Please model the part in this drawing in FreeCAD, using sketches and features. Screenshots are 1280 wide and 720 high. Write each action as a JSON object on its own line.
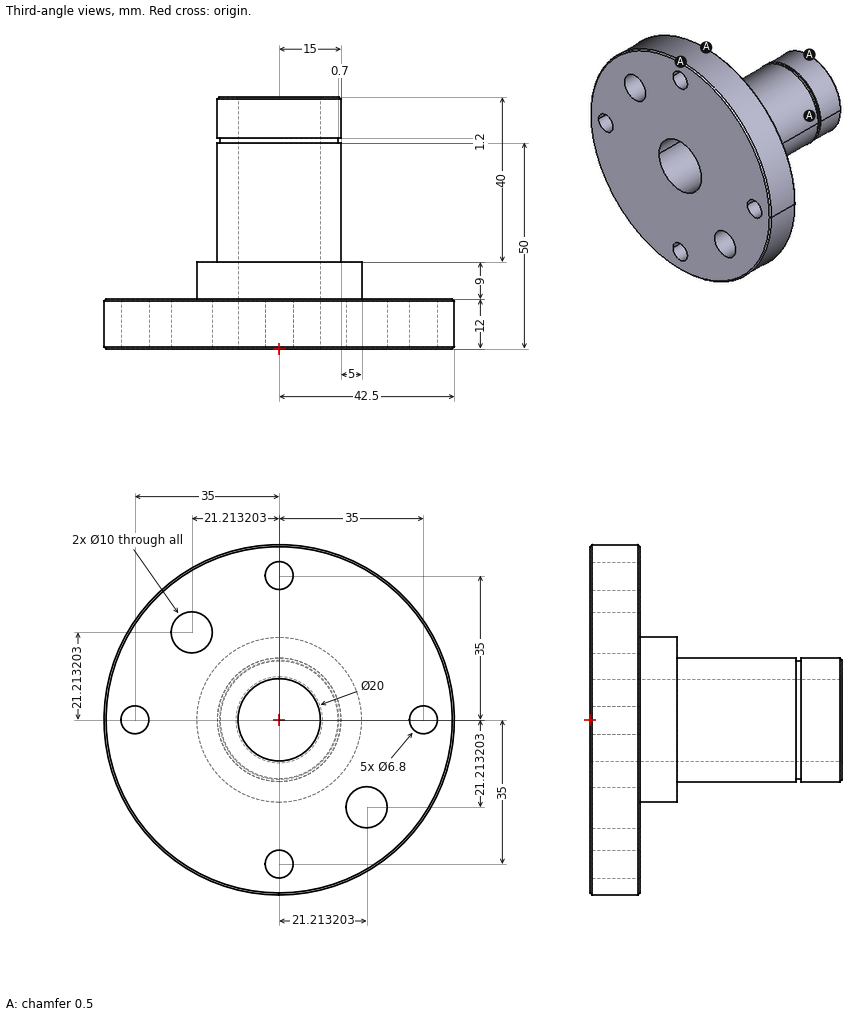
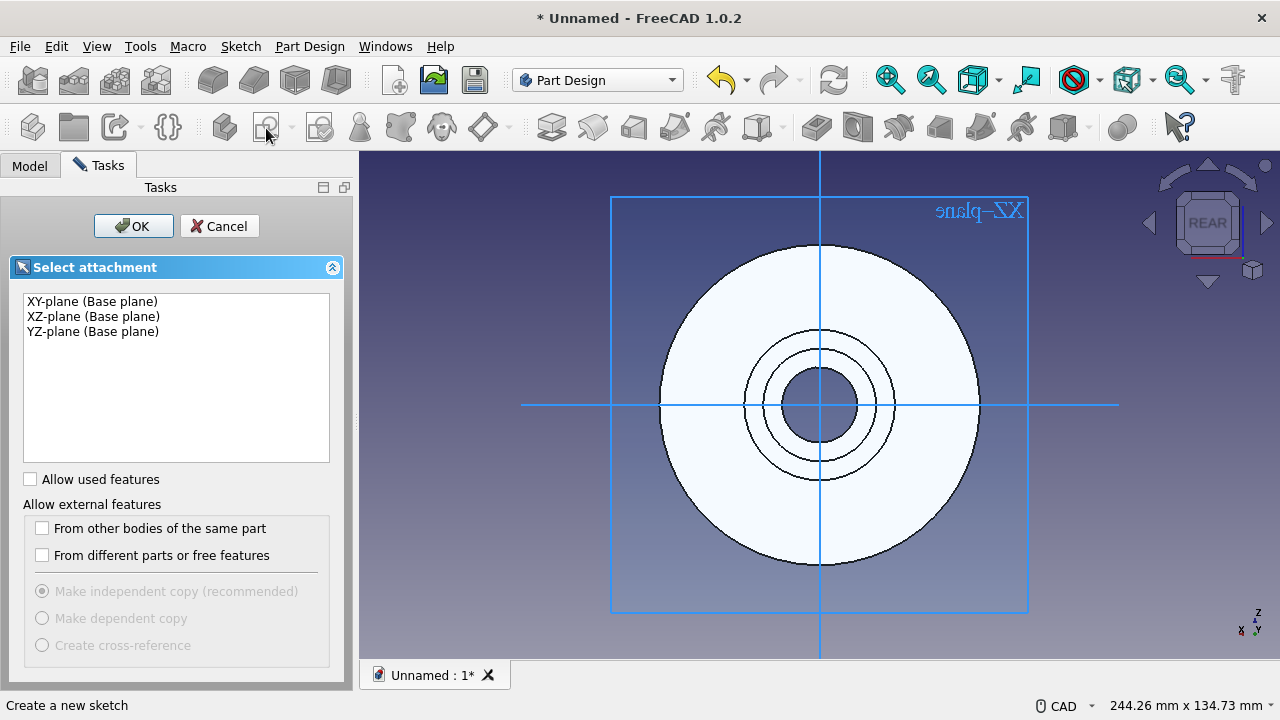
{"action": "left_click", "coordinate": [84, 302]}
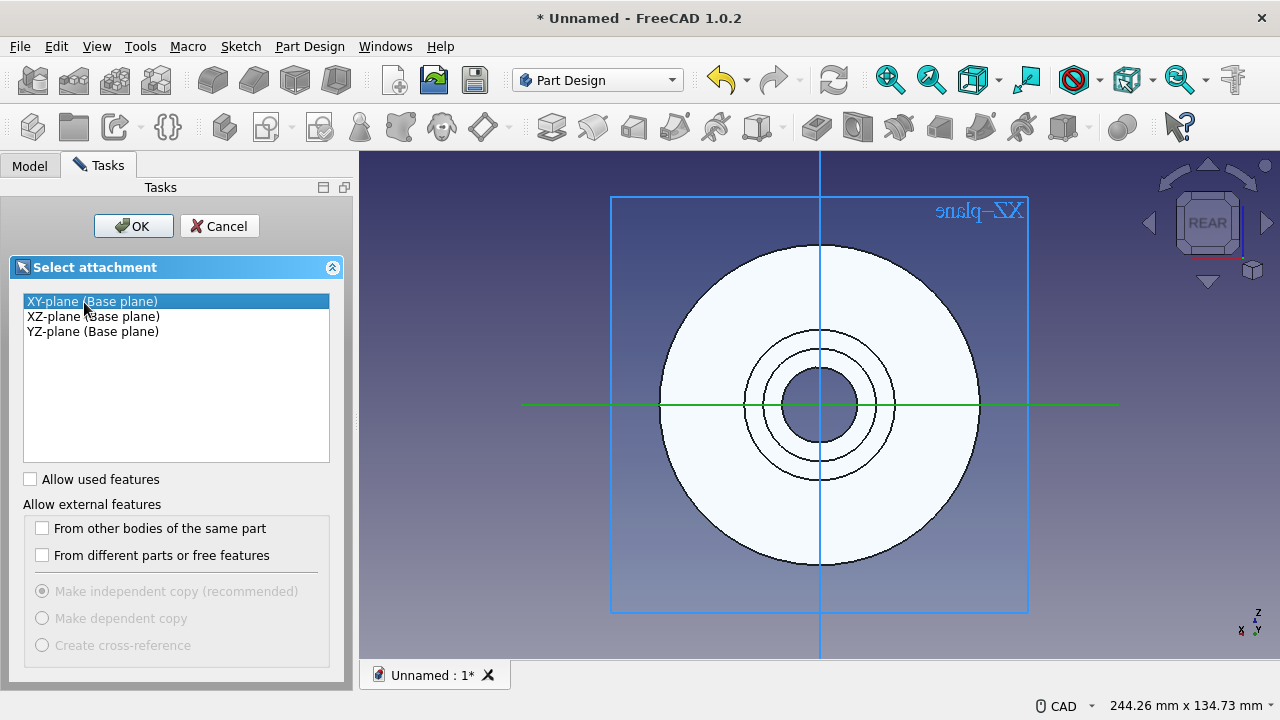
{"action": "left_click", "coordinate": [134, 226]}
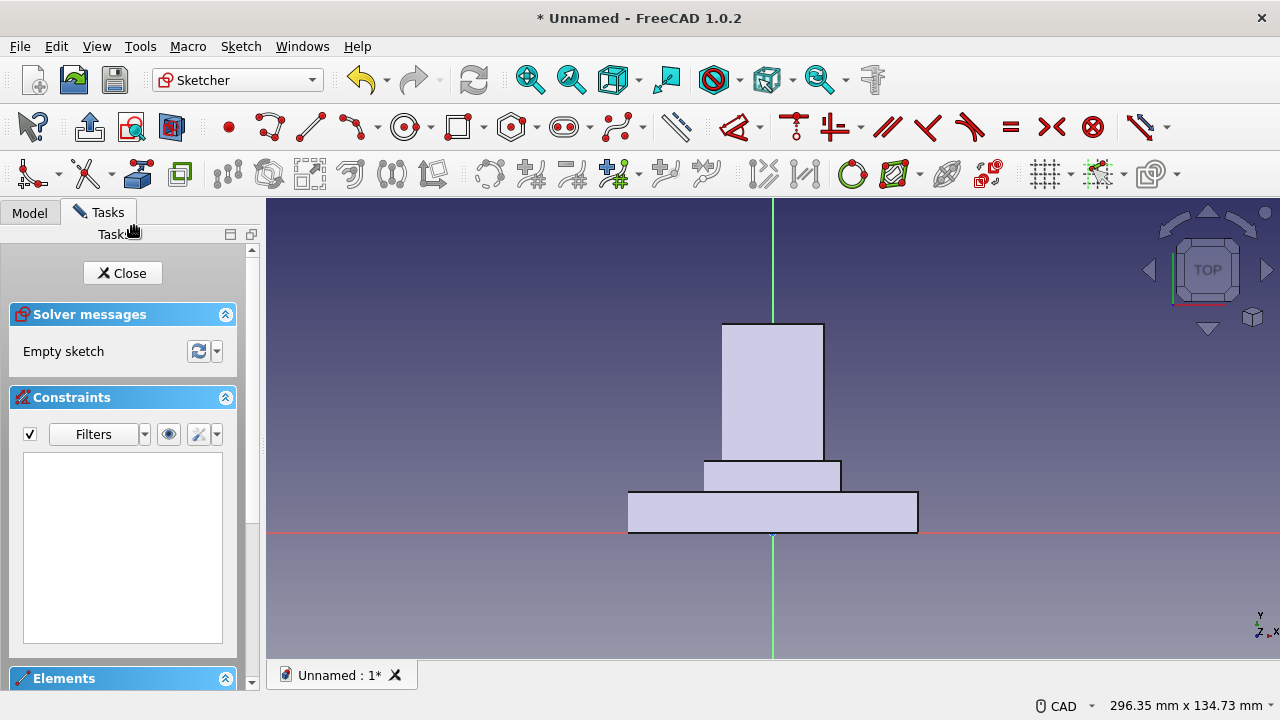
{"action": "left_click", "coordinate": [172, 128]}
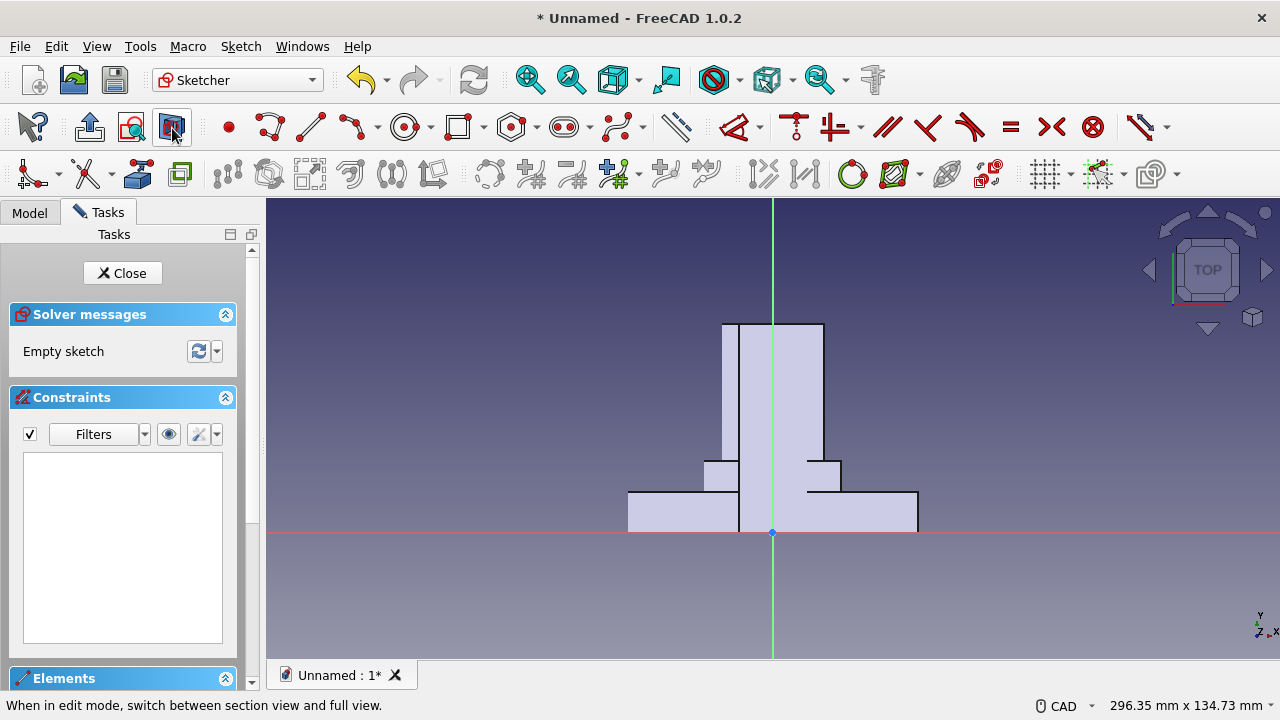
{"action": "scroll", "coordinate": [829, 356], "scroll_direction": "up", "scroll_amount": 15}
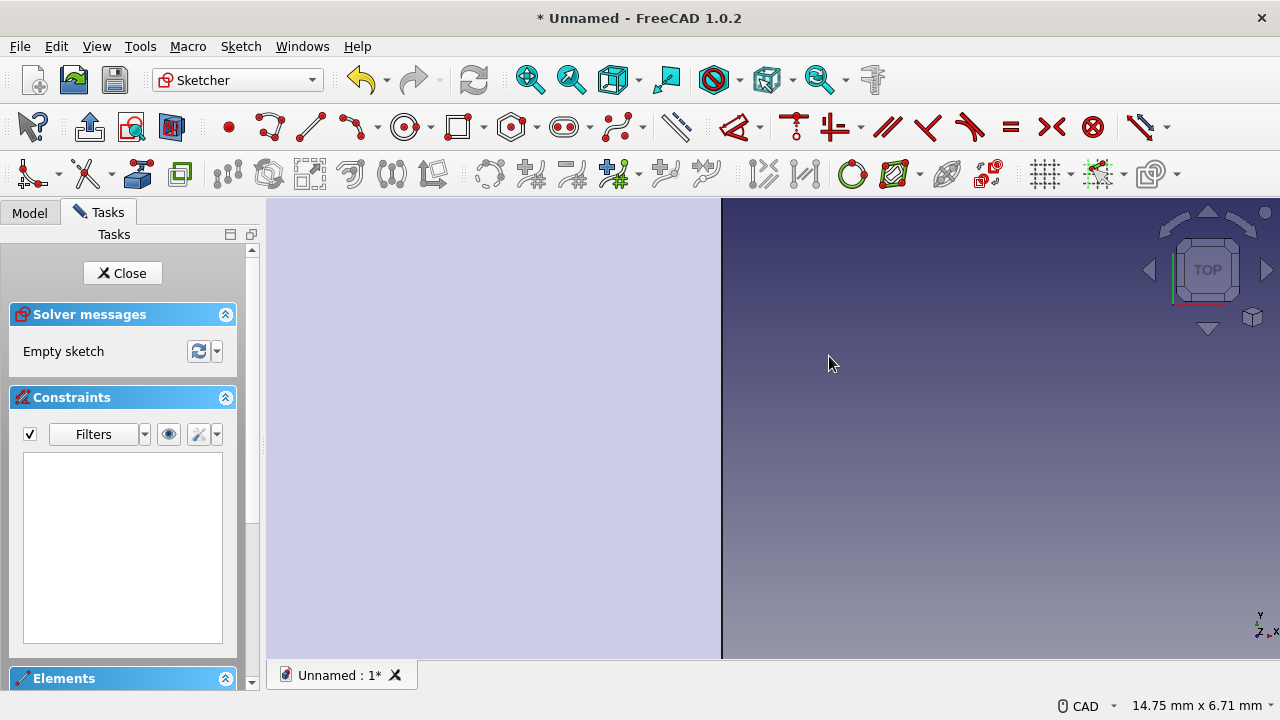
{"action": "scroll", "coordinate": [695, 422], "scroll_direction": "up", "scroll_amount": 6}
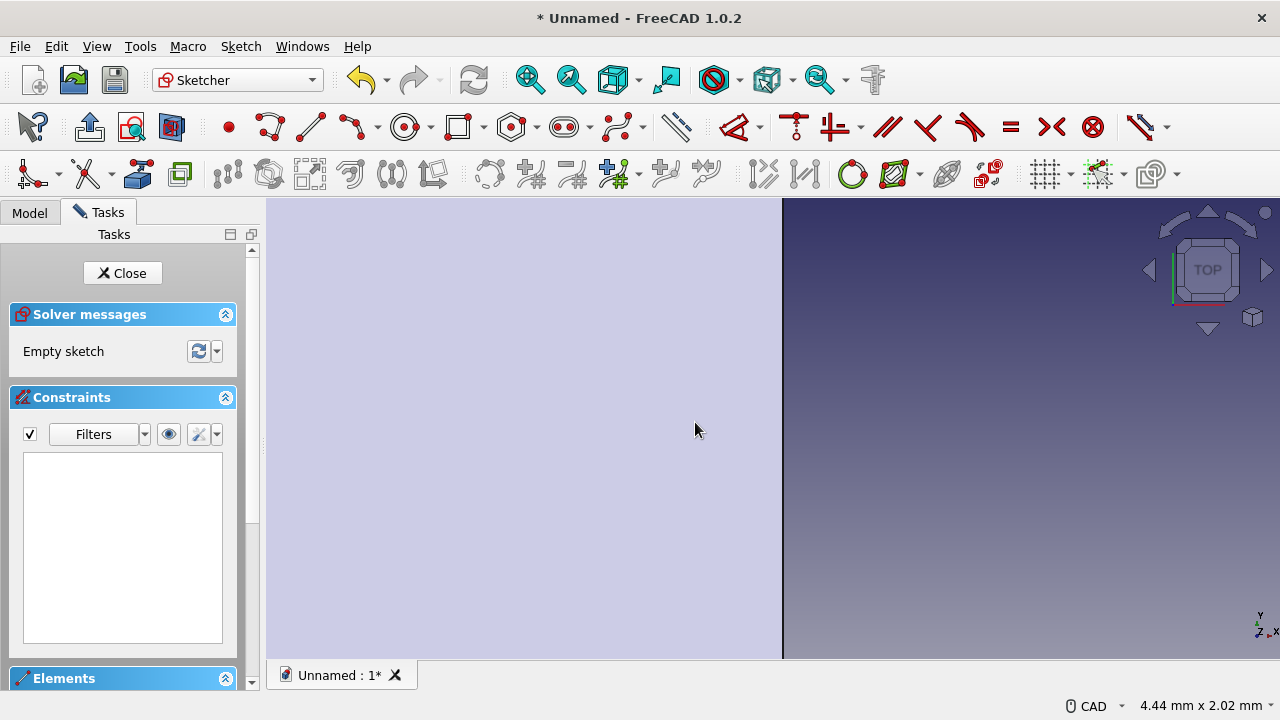
{"action": "key", "text": "g r"}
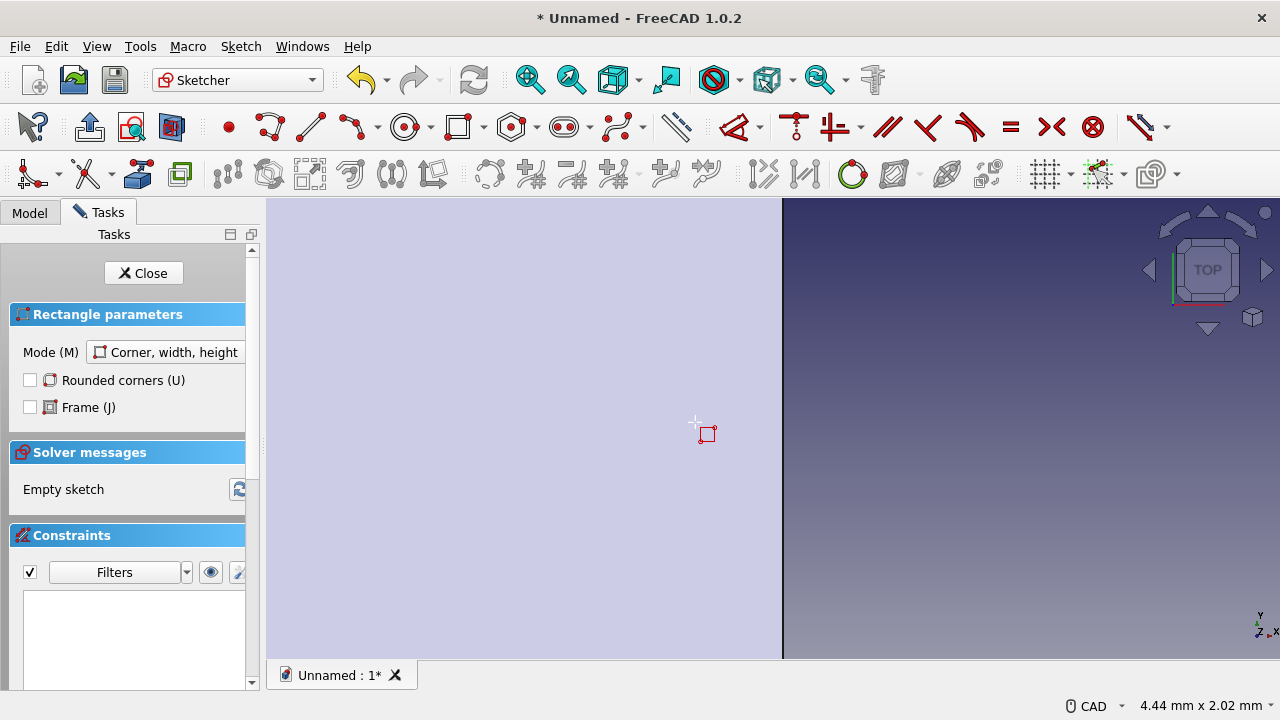
{"action": "left_click", "coordinate": [624, 291]}
{"action": "left_click", "coordinate": [783, 565]}
{"action": "key", "text": "Escape"}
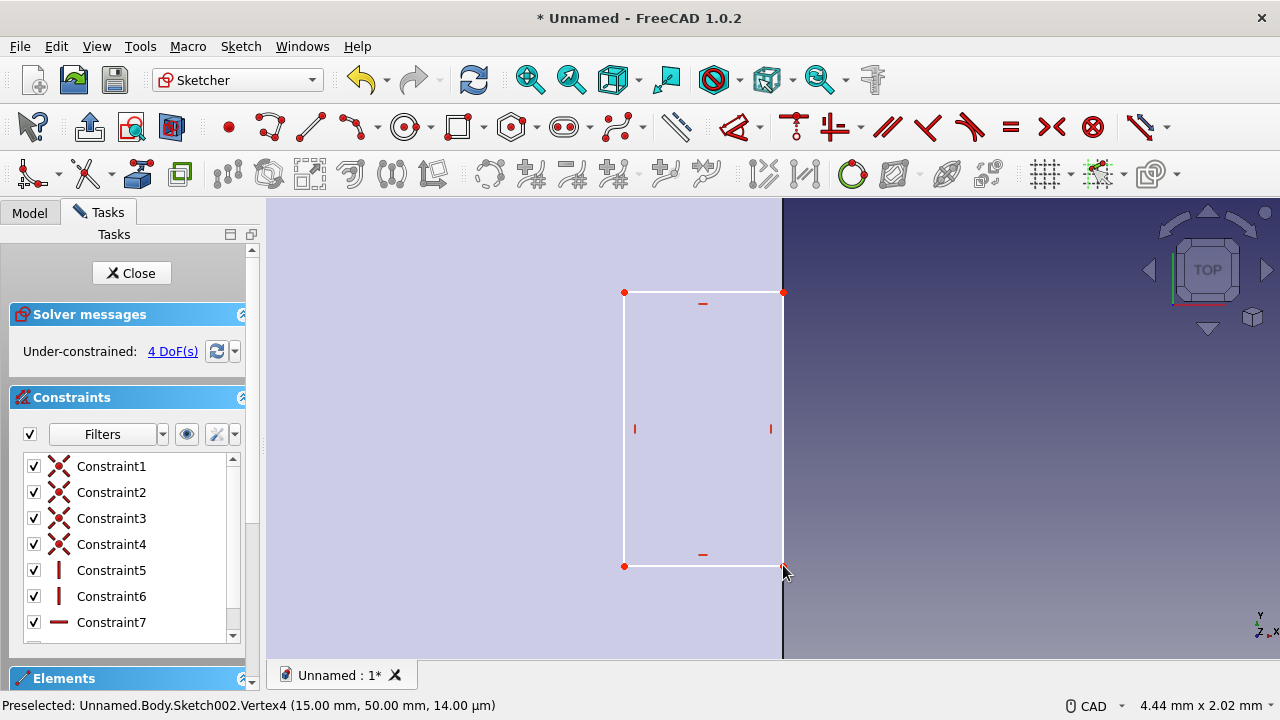
{"action": "left_click", "coordinate": [734, 128]}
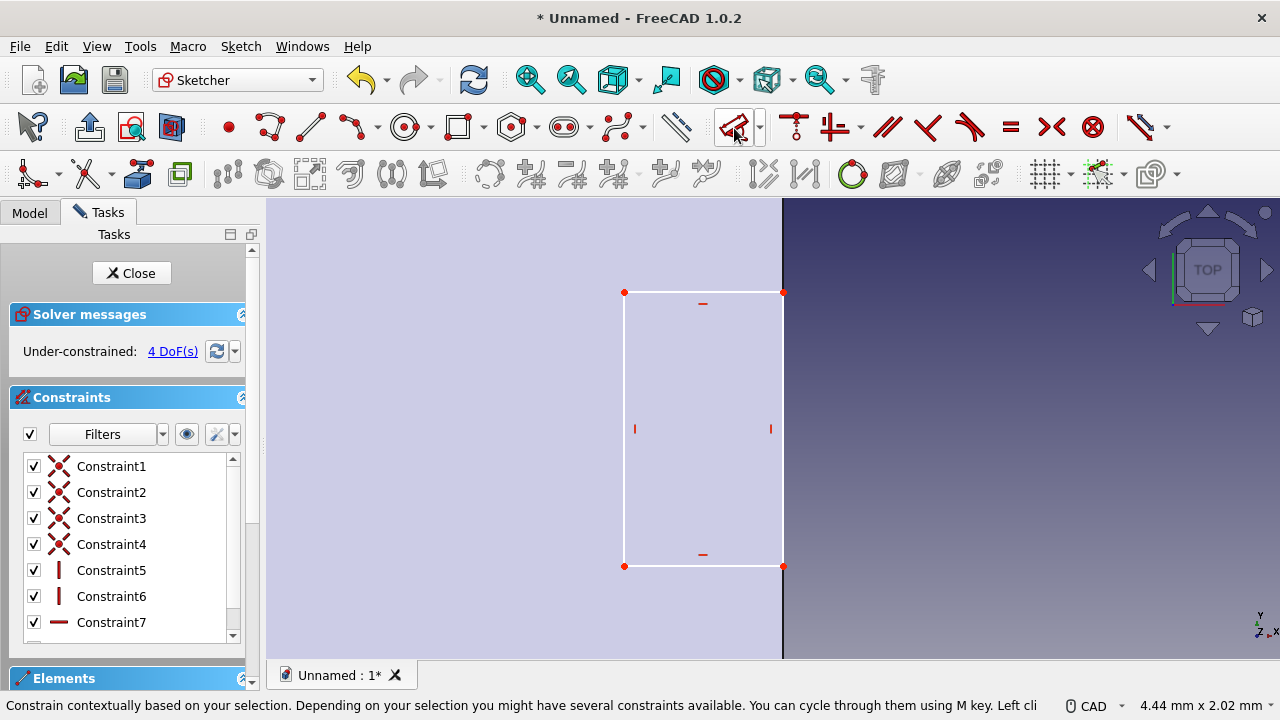
{"action": "left_click", "coordinate": [624, 374]}
{"action": "left_click", "coordinate": [590, 429]}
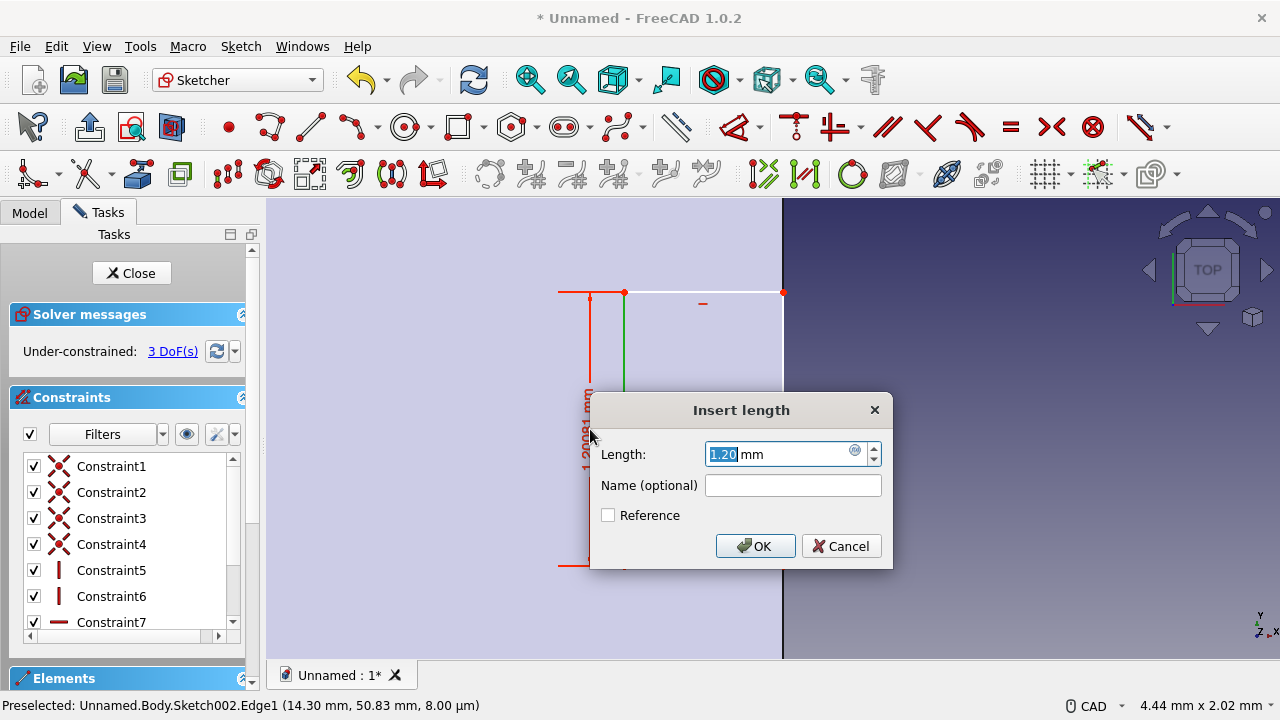
{"action": "type", "text": "1.2"}
{"action": "key", "text": "Return"}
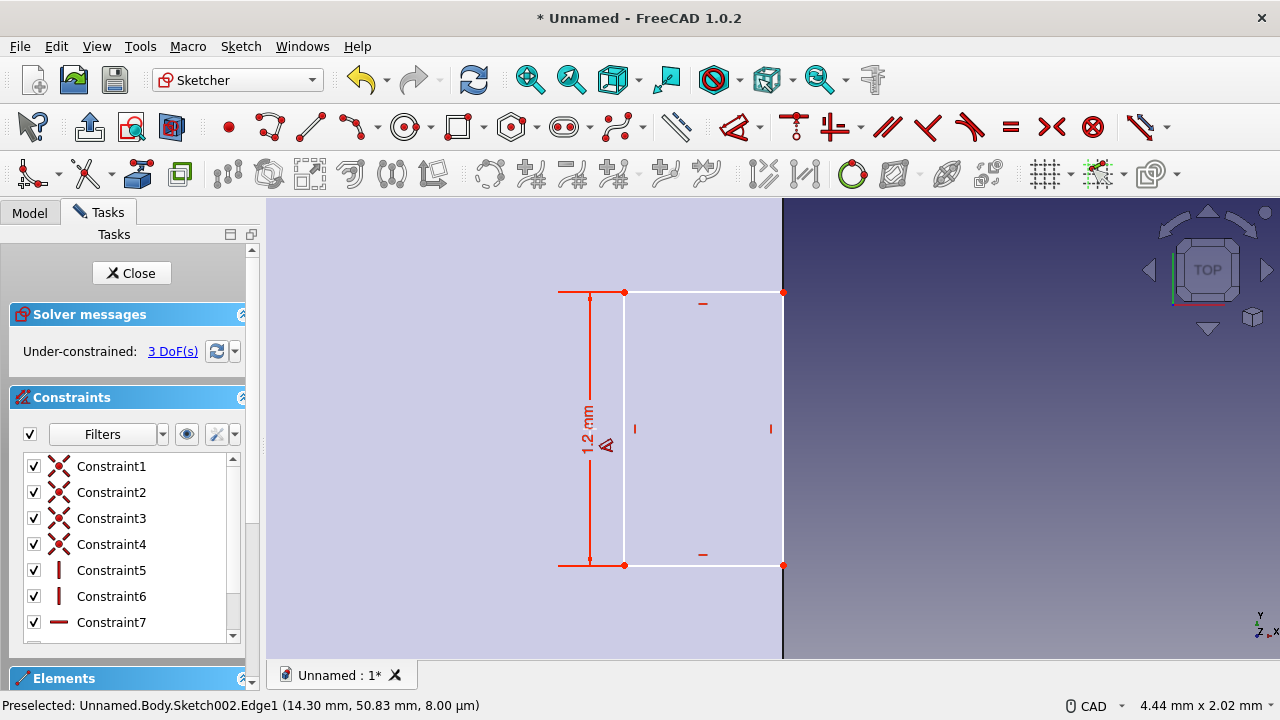
{"action": "left_click", "coordinate": [672, 566]}
{"action": "left_click", "coordinate": [704, 600]}